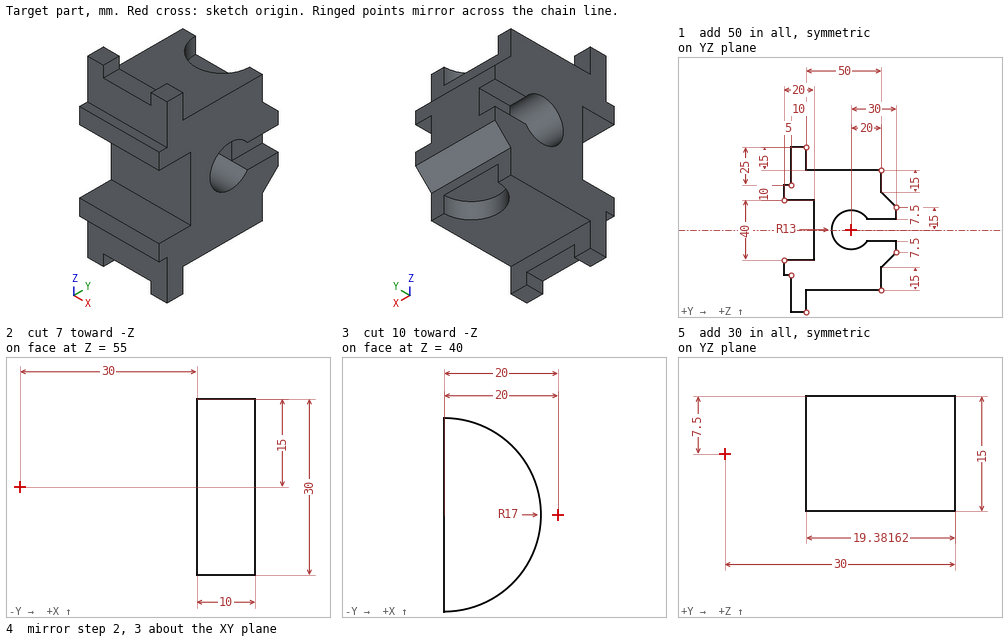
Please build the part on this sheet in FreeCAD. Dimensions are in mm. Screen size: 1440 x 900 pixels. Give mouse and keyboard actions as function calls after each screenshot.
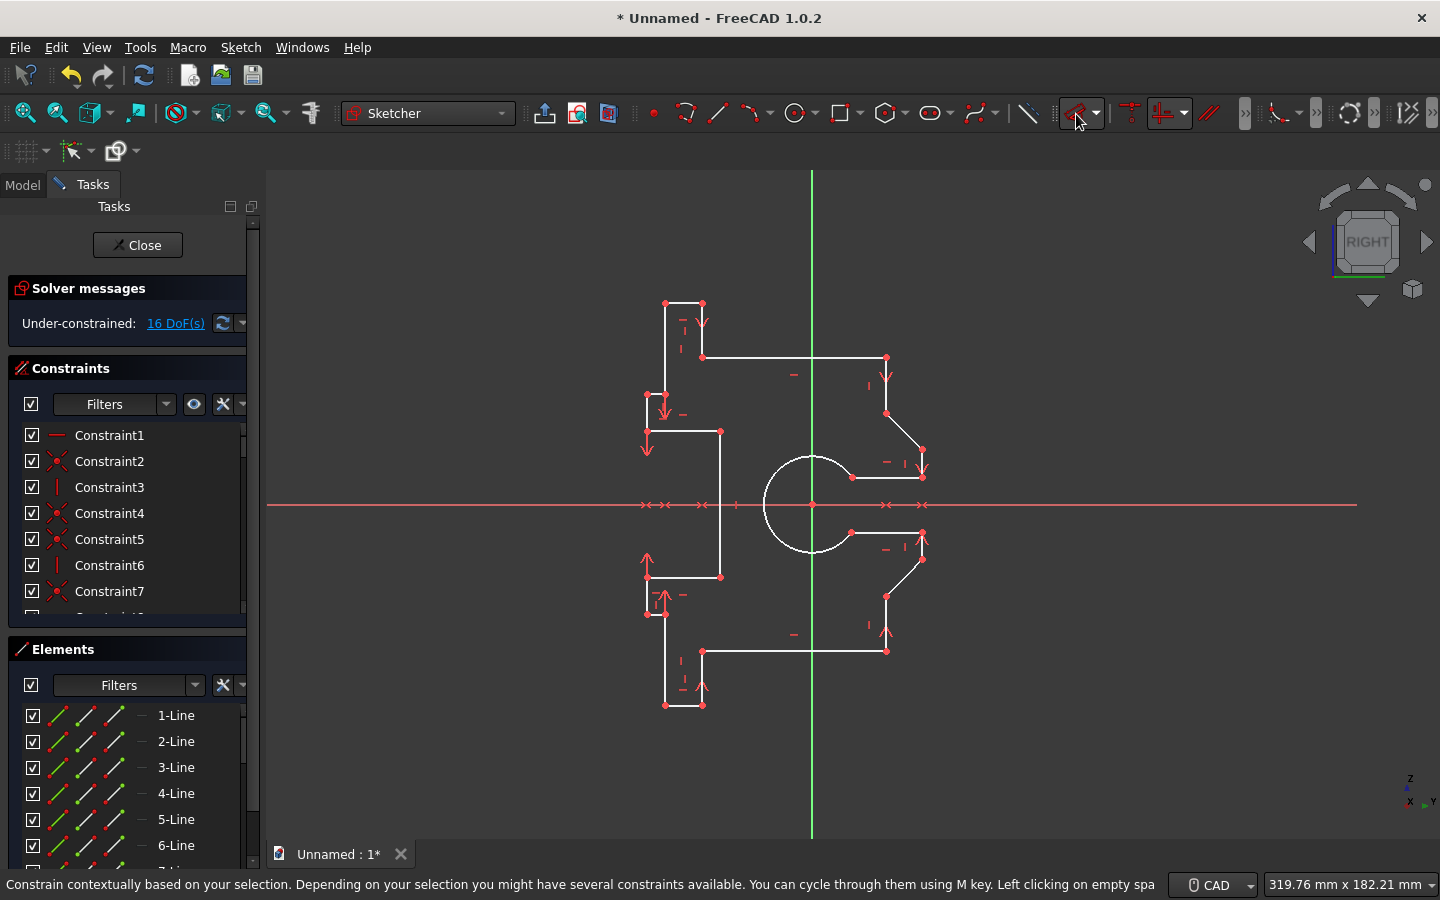
click(788, 463)
click(772, 435)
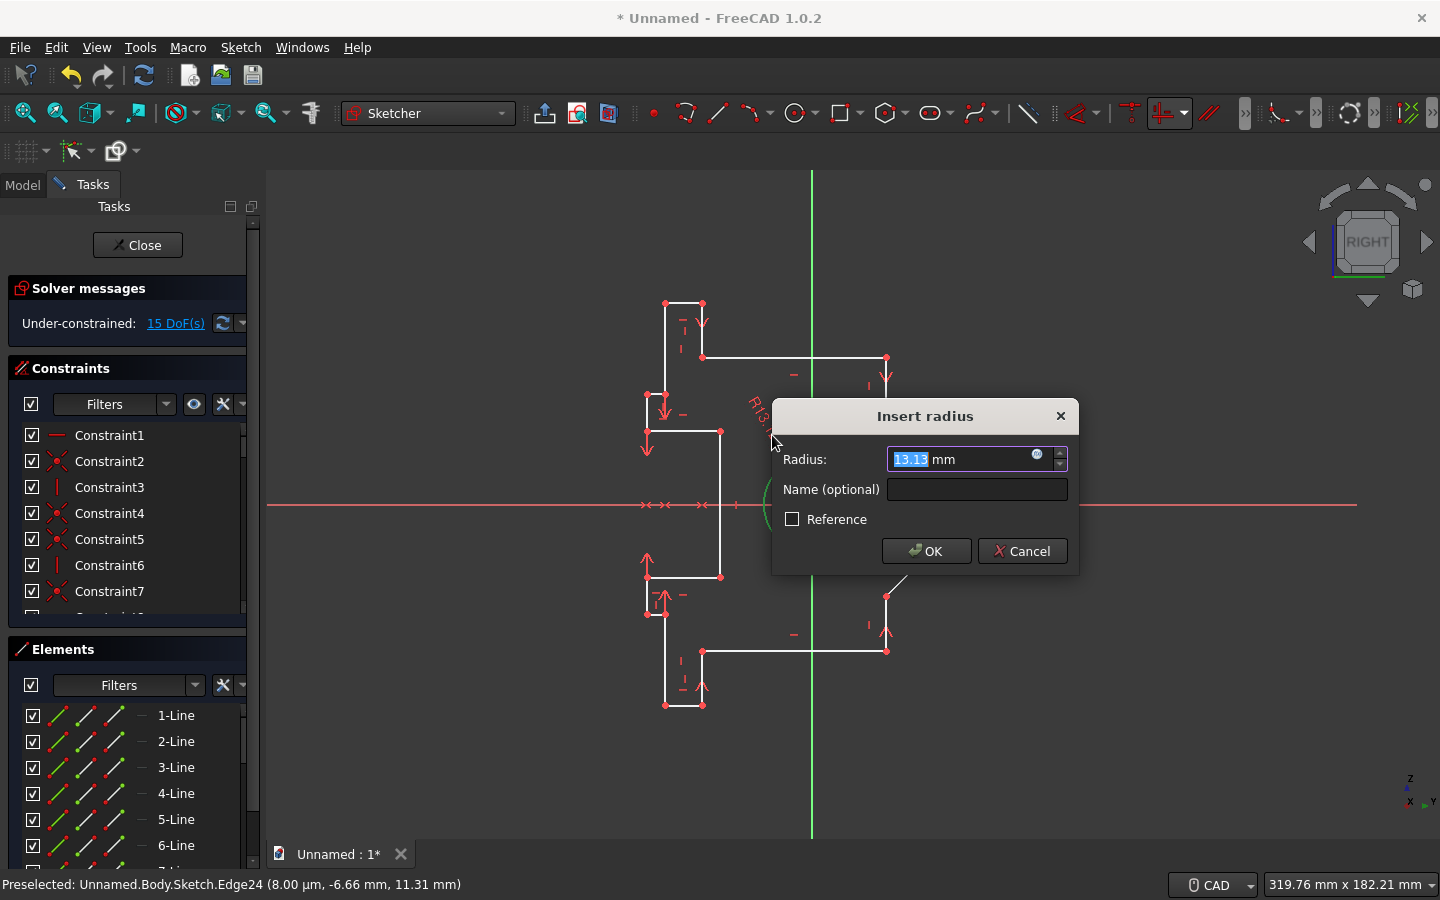
text(13)
key(Return)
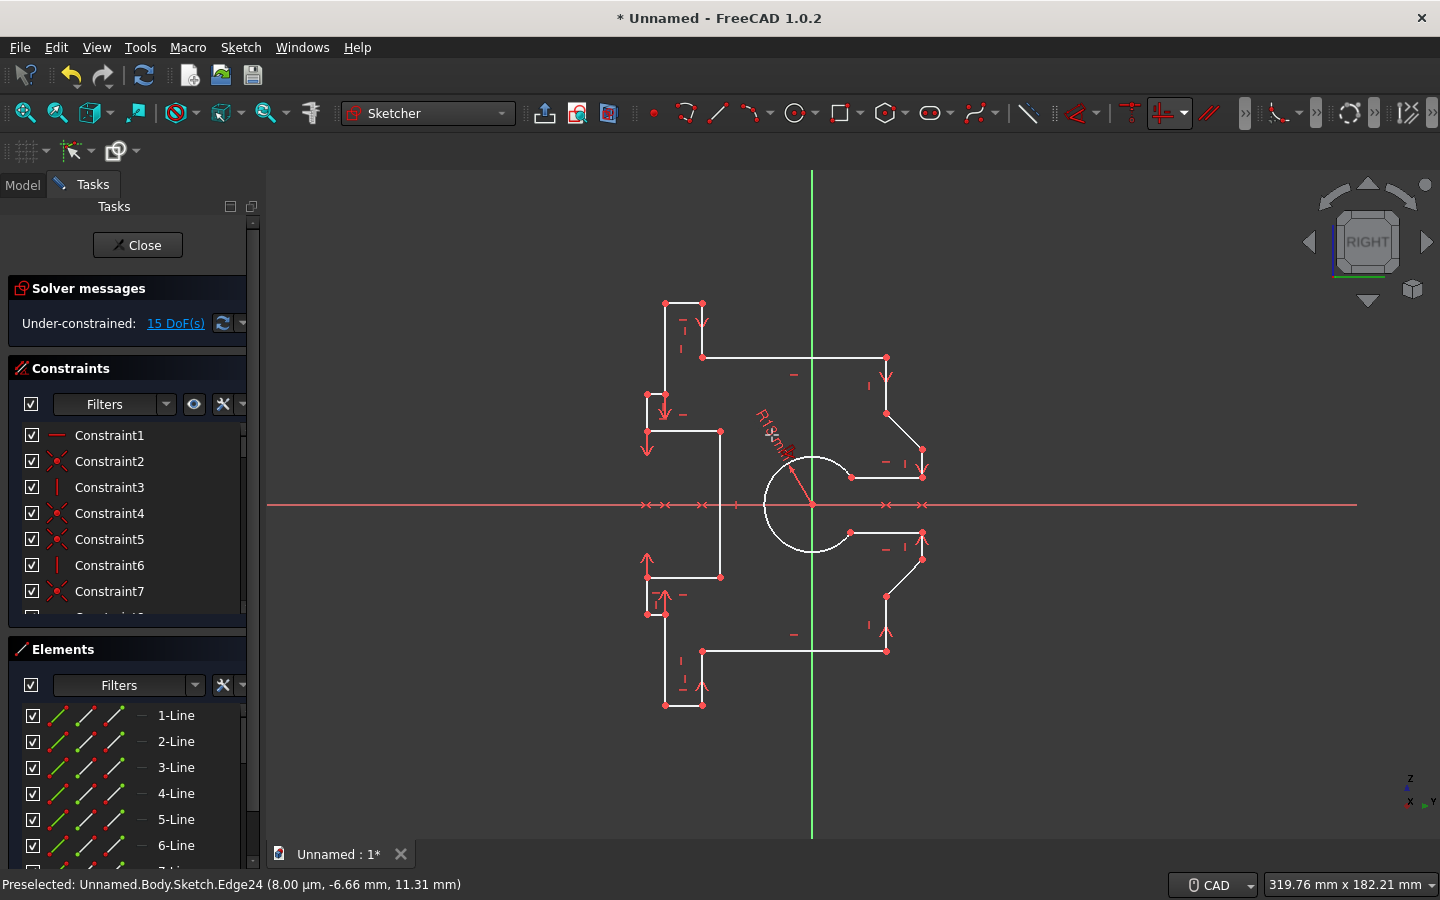
scroll(656, 394, up, 4)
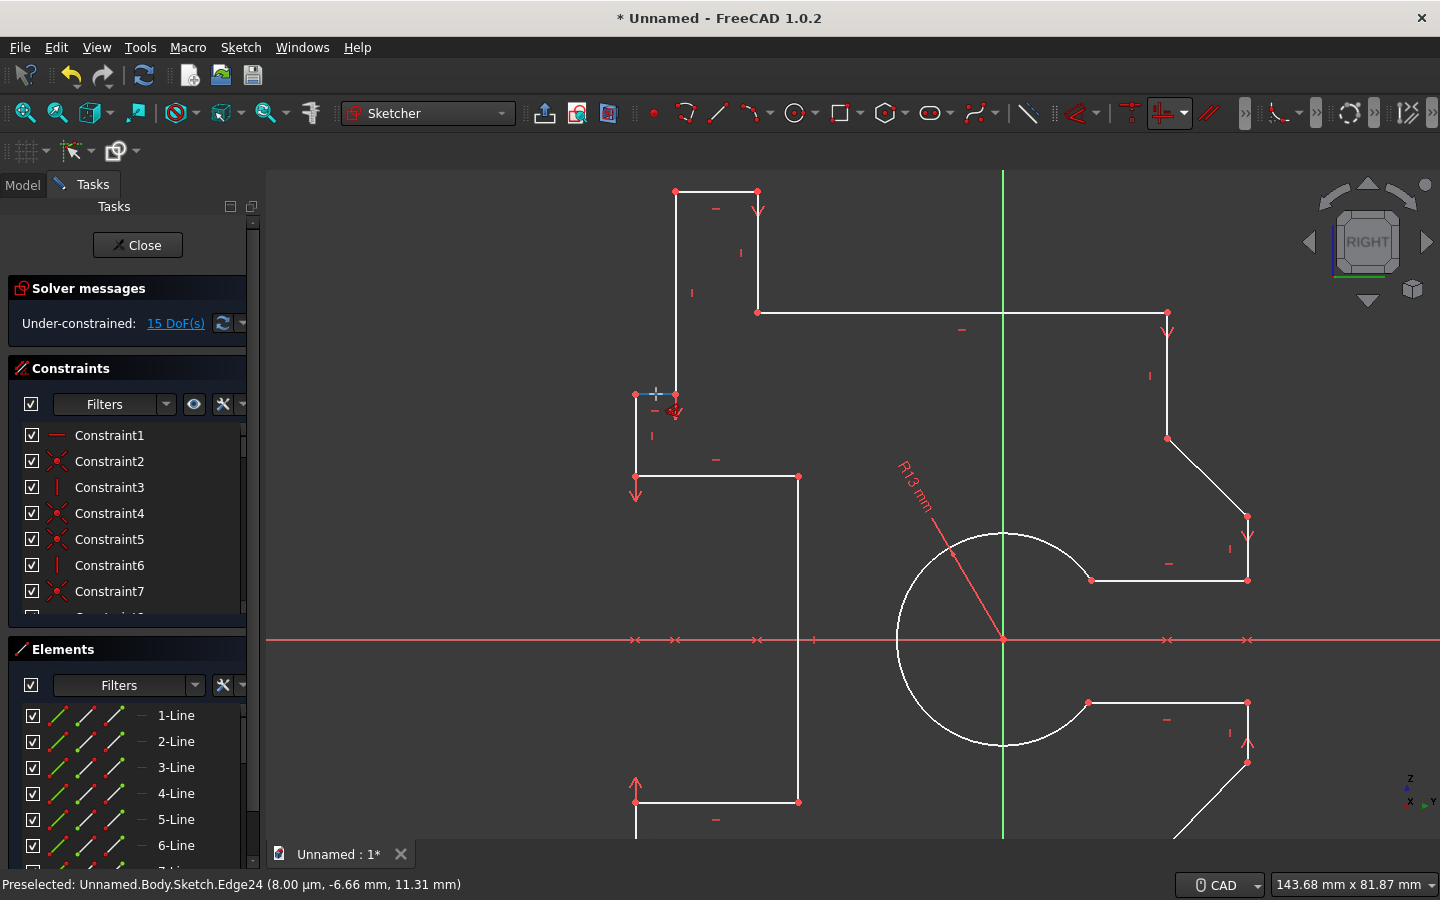
click(656, 394)
click(656, 360)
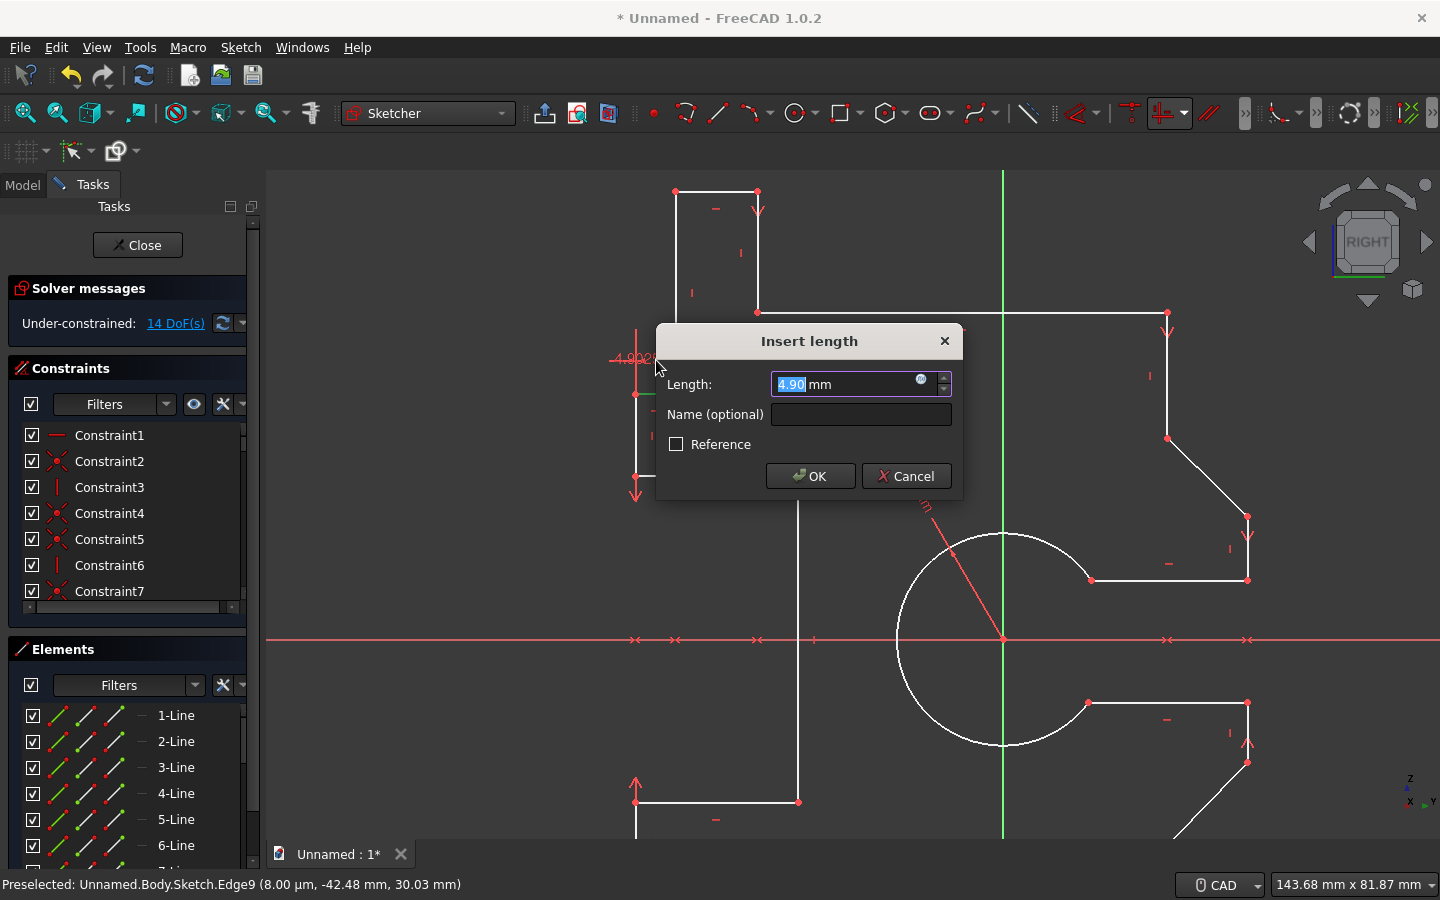
text(5)
key(Return)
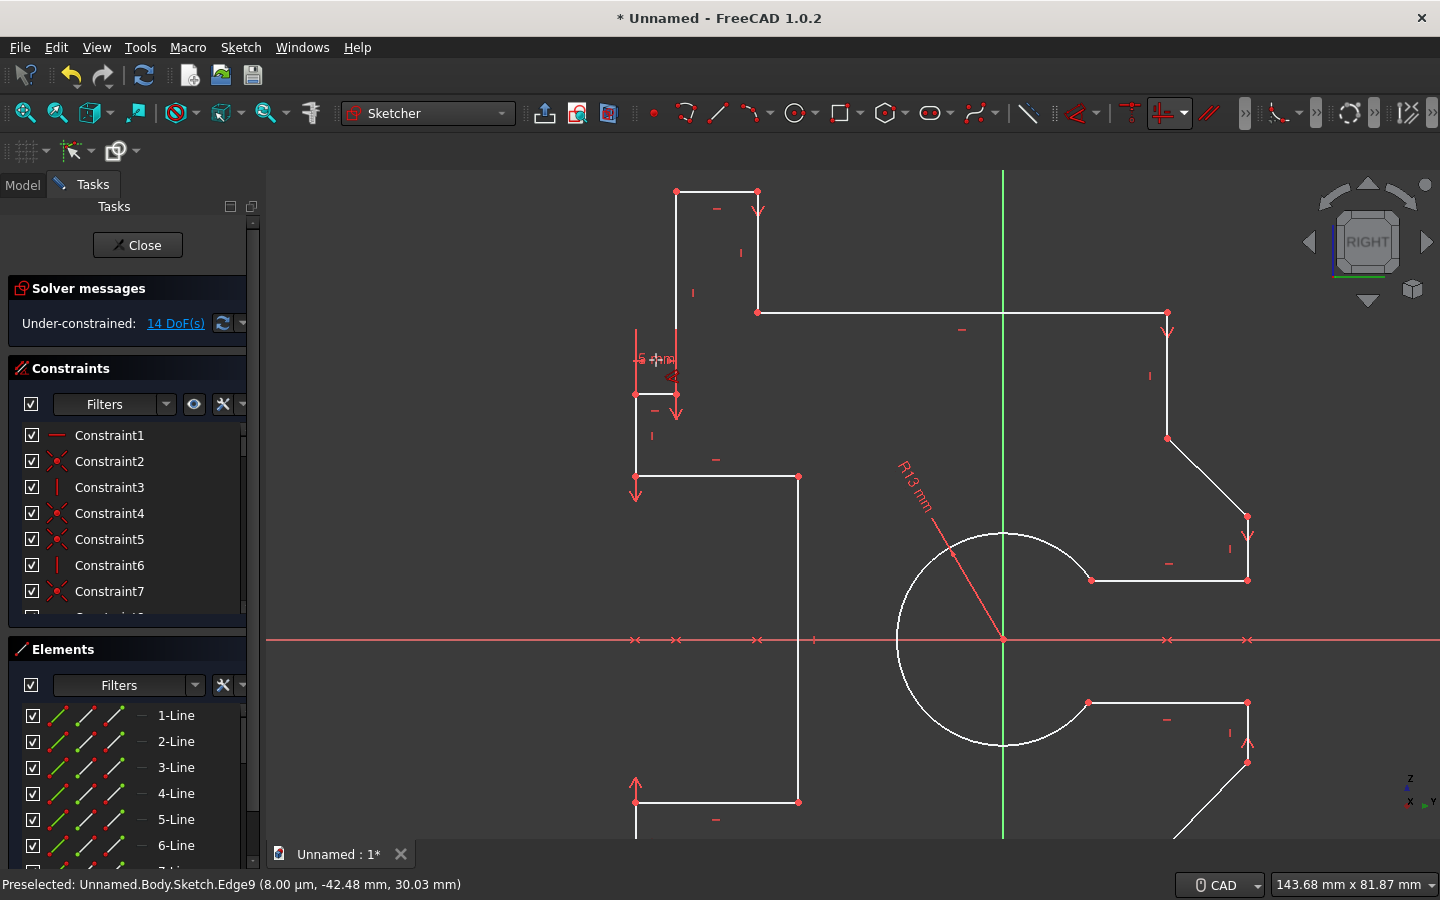
click(1167, 401)
click(1201, 376)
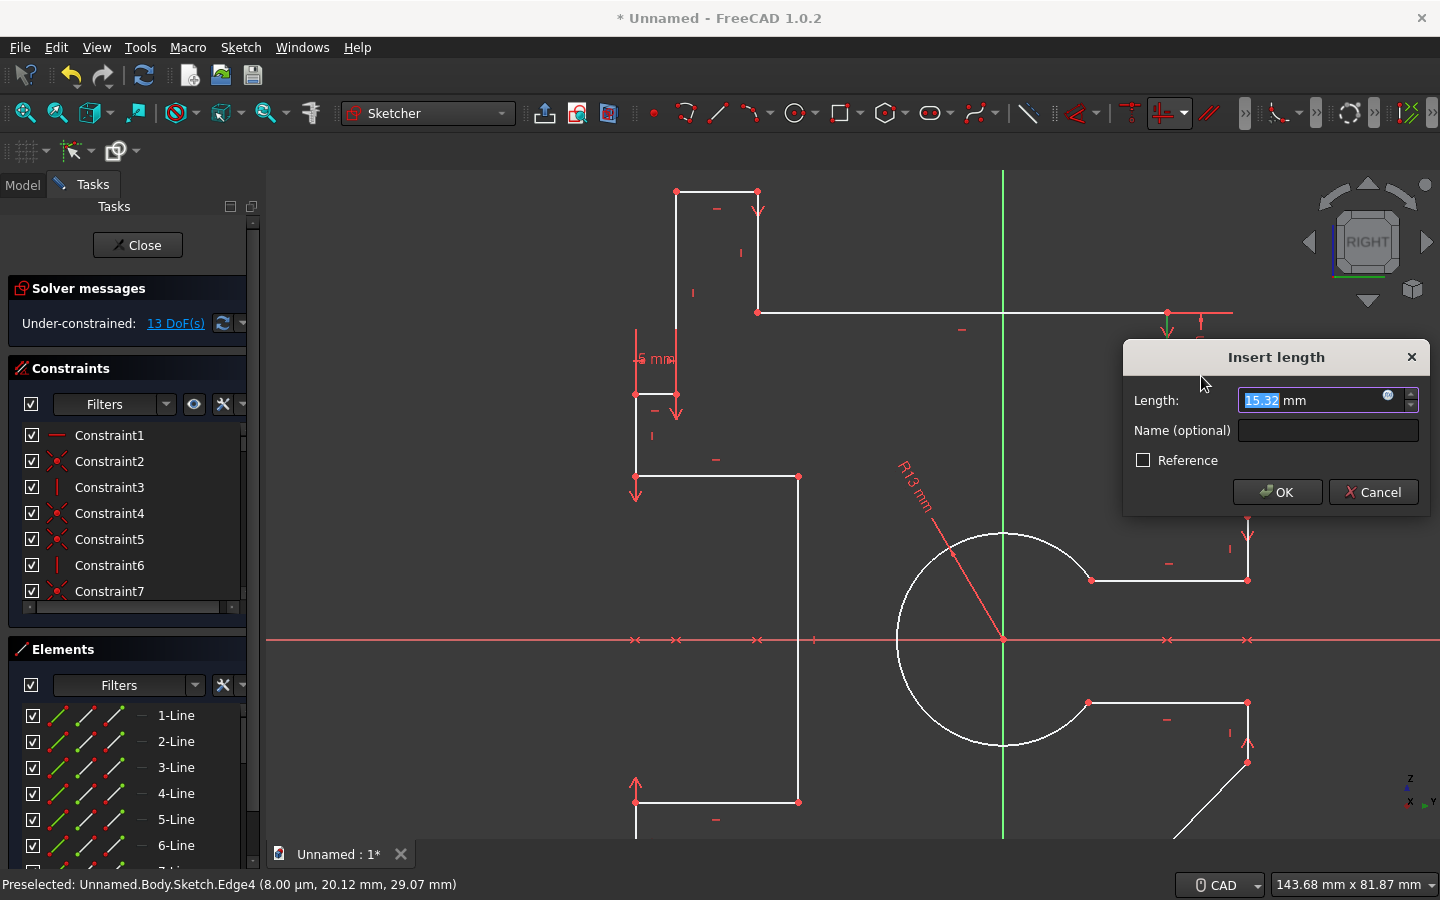
text(15)
key(Return)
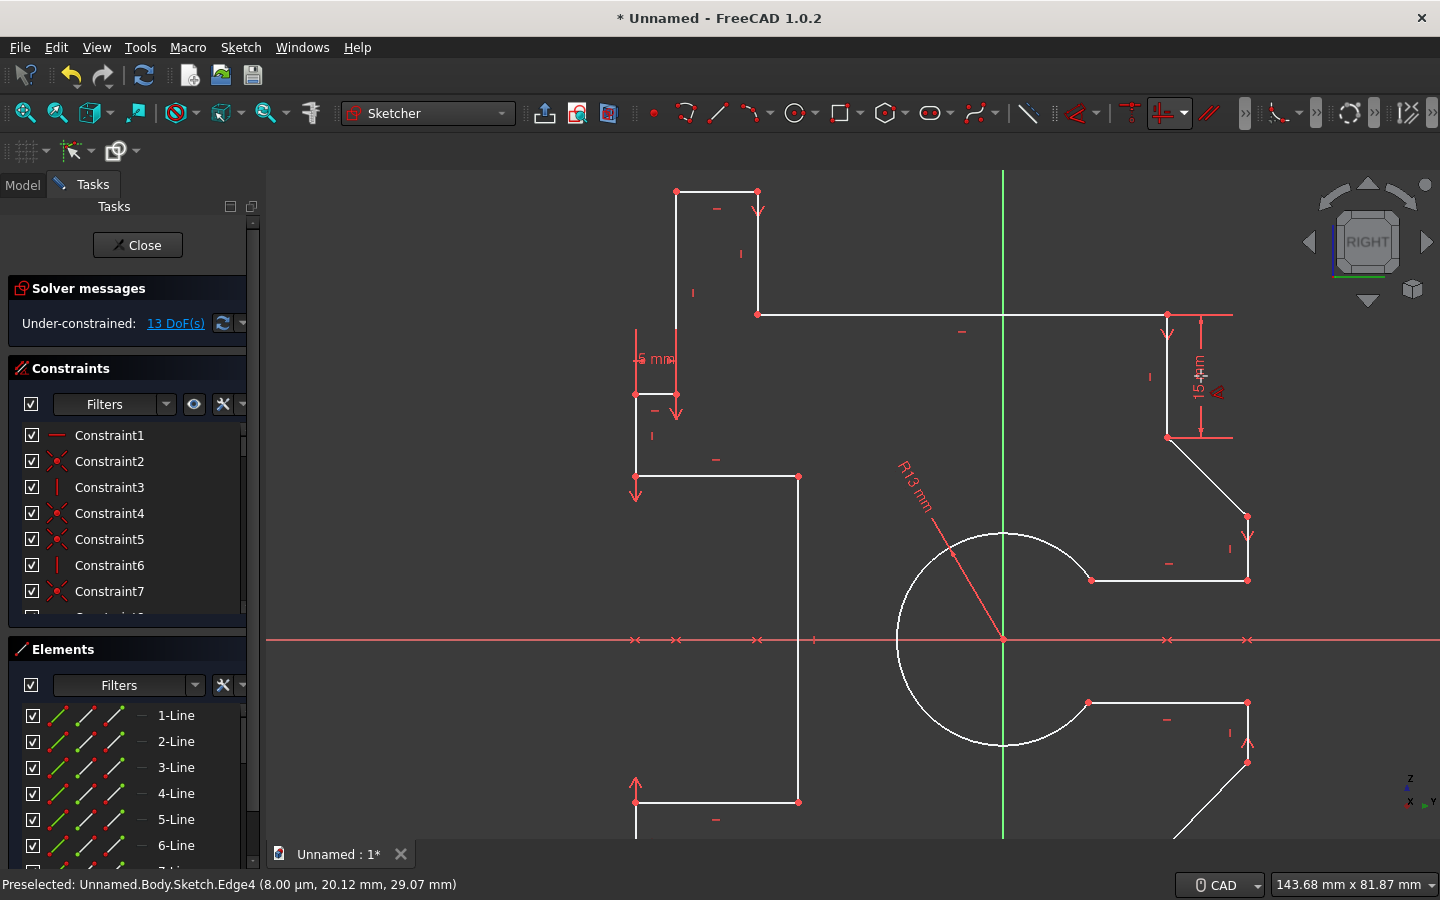
click(1045, 315)
click(963, 281)